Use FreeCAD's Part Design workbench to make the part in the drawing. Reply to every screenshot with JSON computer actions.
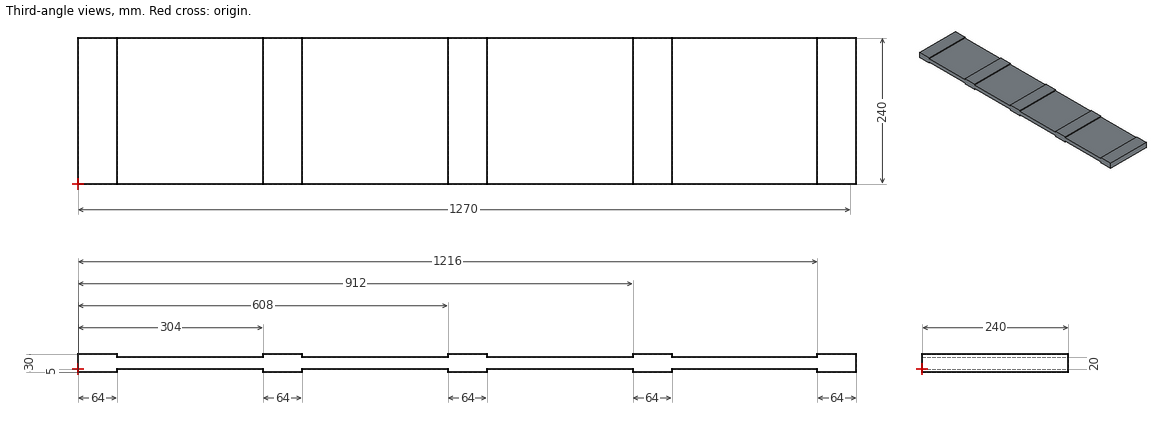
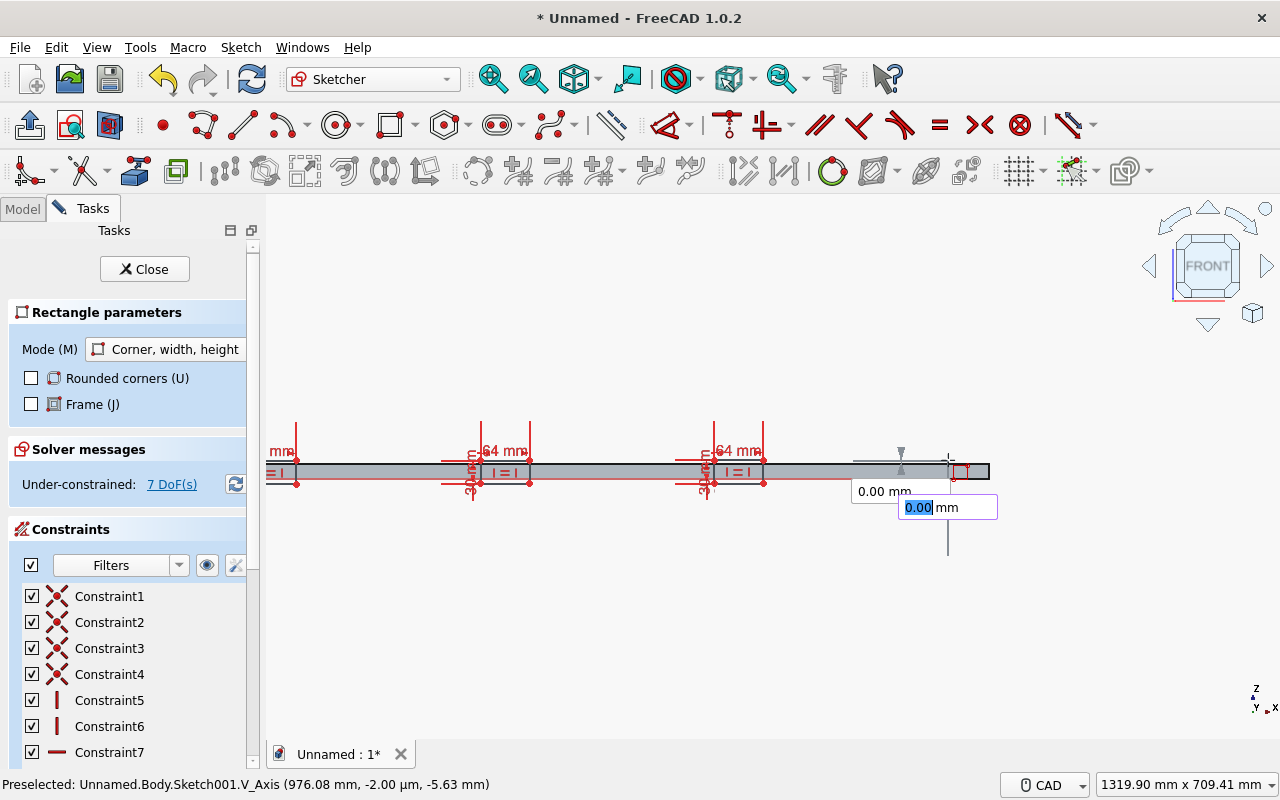
{"action": "scroll", "coordinate": [997, 483], "scroll_direction": "up", "scroll_amount": 8}
{"action": "mouse_move", "coordinate": [994, 481]}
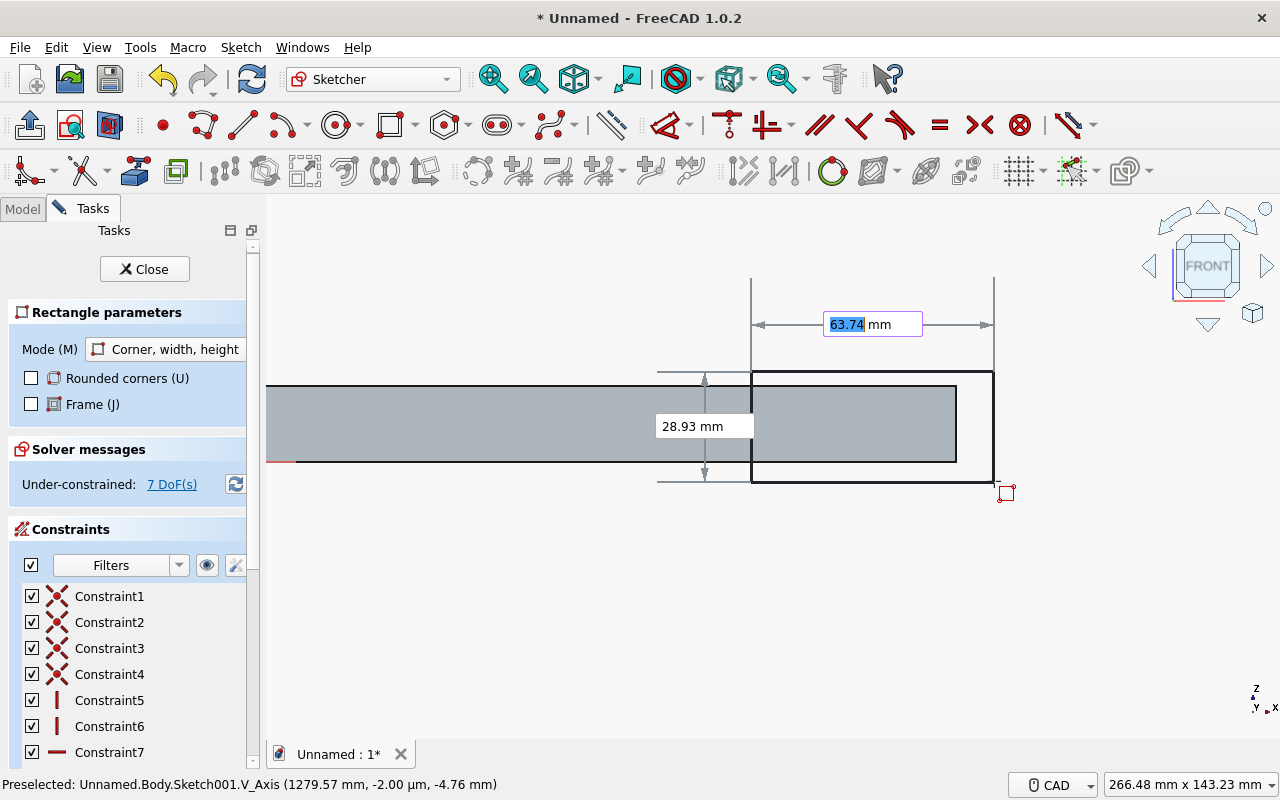
{"action": "type", "text": "64"}
{"action": "key", "text": "Tab"}
{"action": "type", "text": "30"}
{"action": "key", "text": "Return"}
{"action": "key", "text": "Escape"}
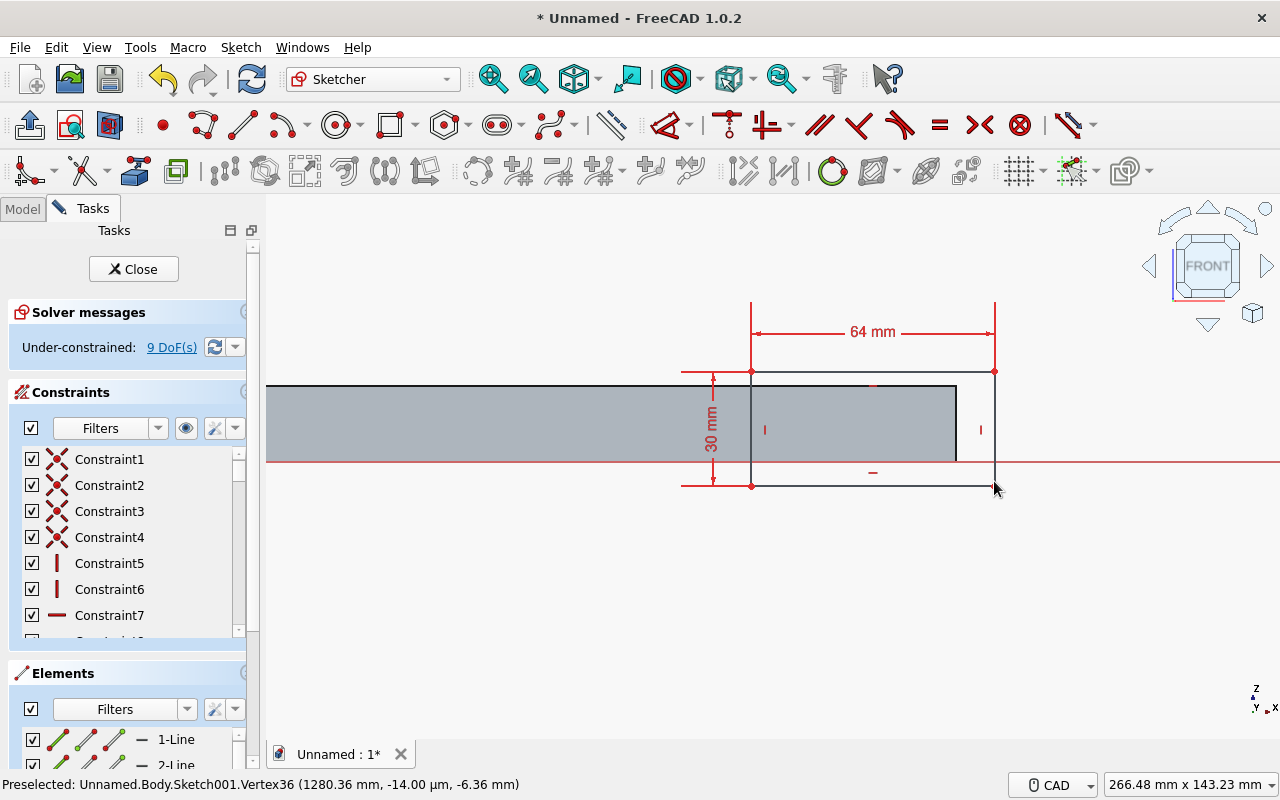
{"action": "key", "text": "d"}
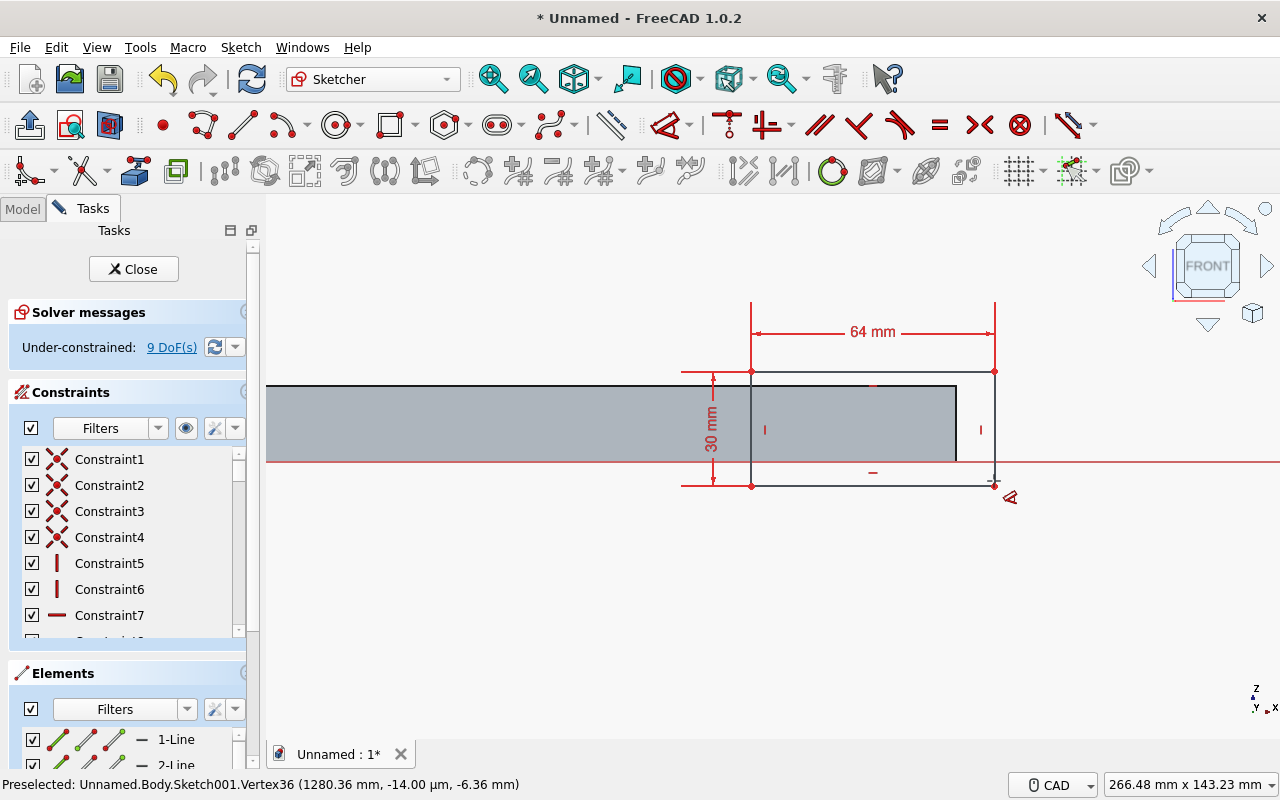
{"action": "scroll", "coordinate": [972, 472], "scroll_direction": "down", "scroll_amount": 11}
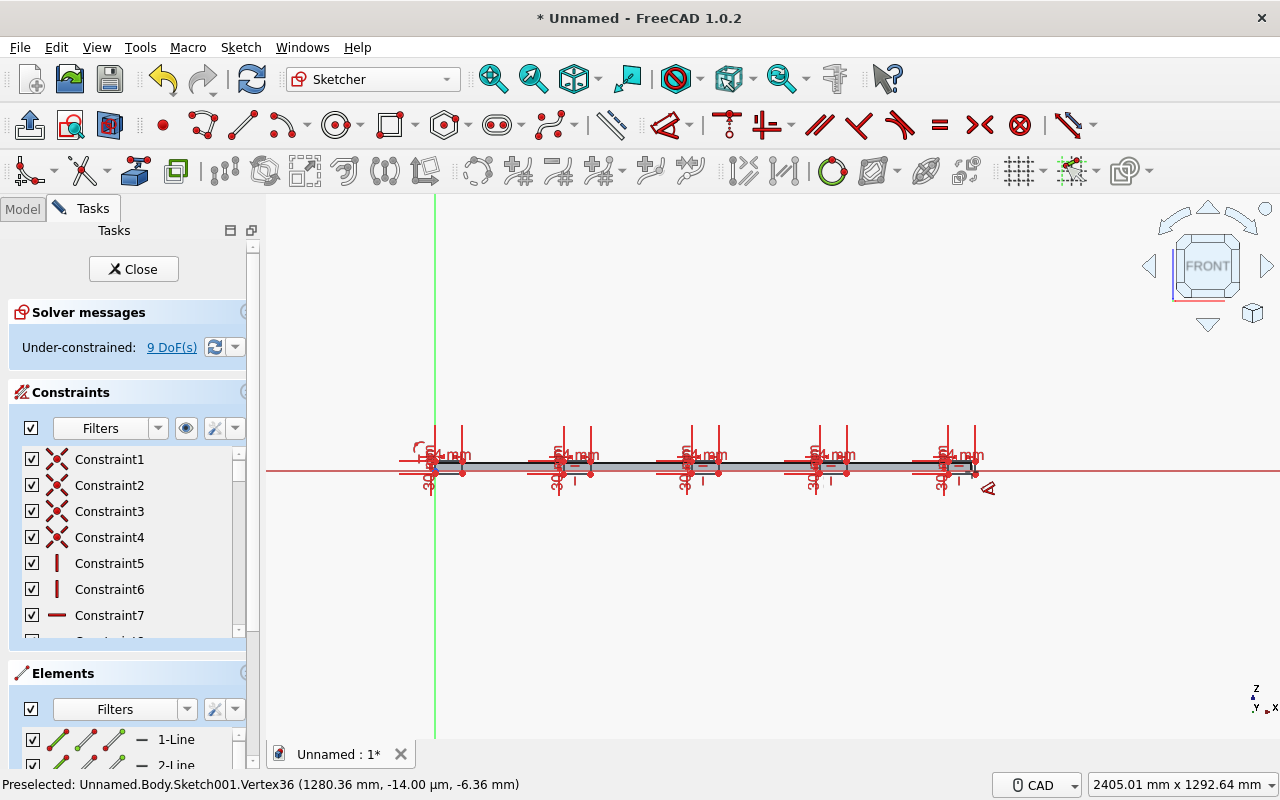
{"action": "scroll", "coordinate": [435, 474], "scroll_direction": "up", "scroll_amount": 15}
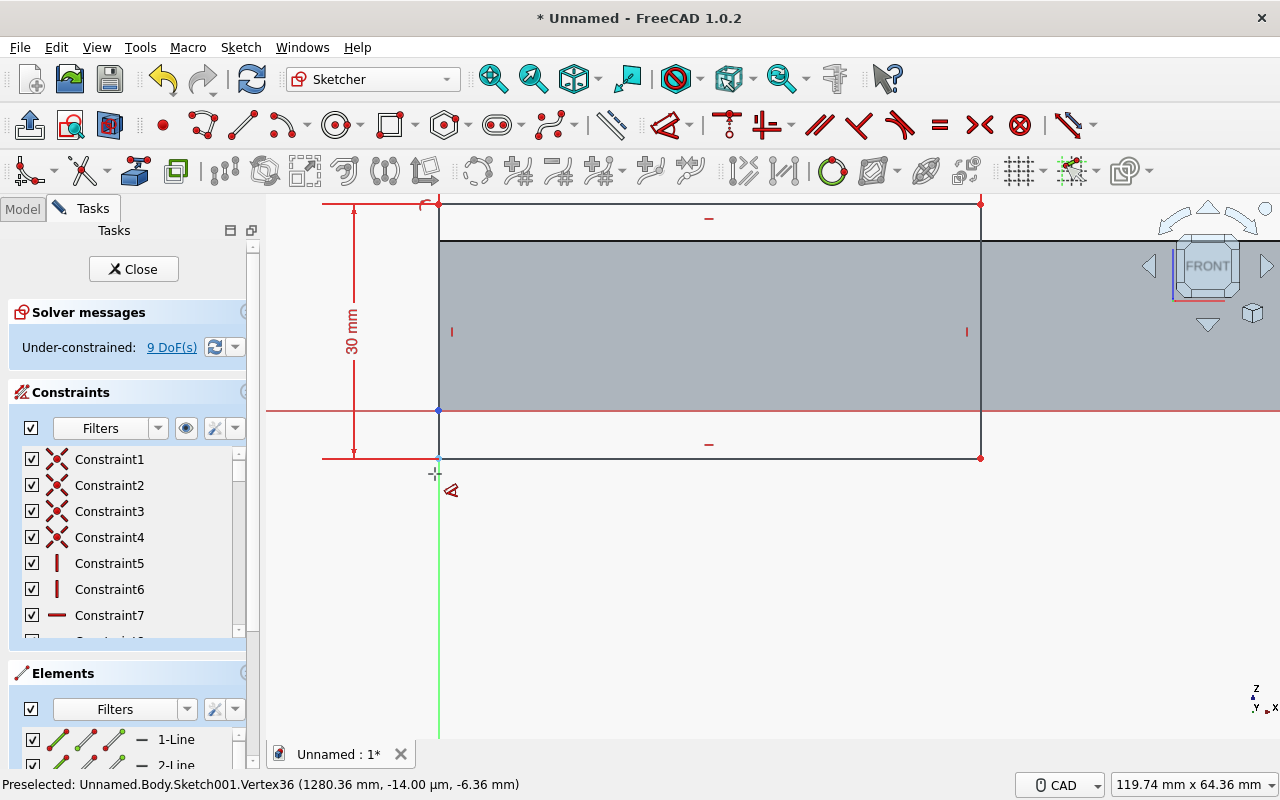
{"action": "left_click", "coordinate": [439, 459]}
{"action": "left_click", "coordinate": [405, 435]}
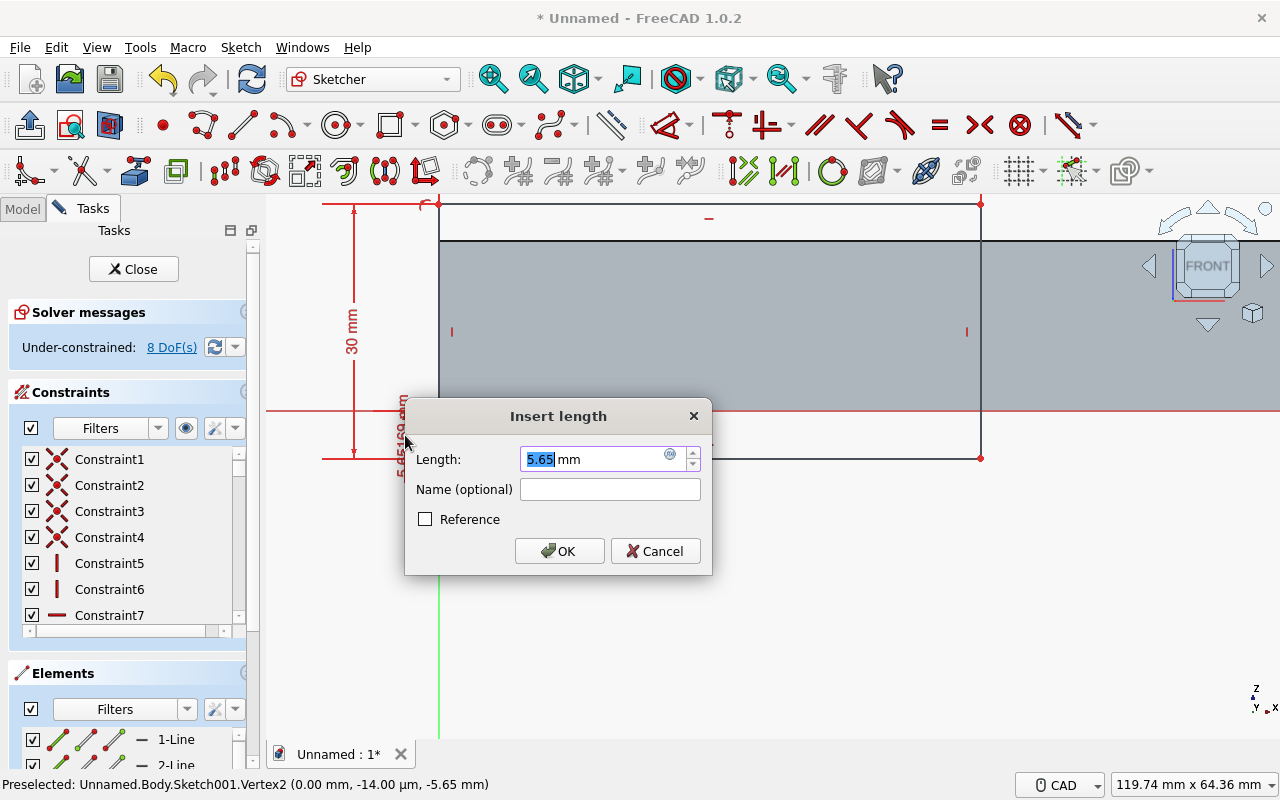
{"action": "type", "text": "5"}
{"action": "key", "text": "Return"}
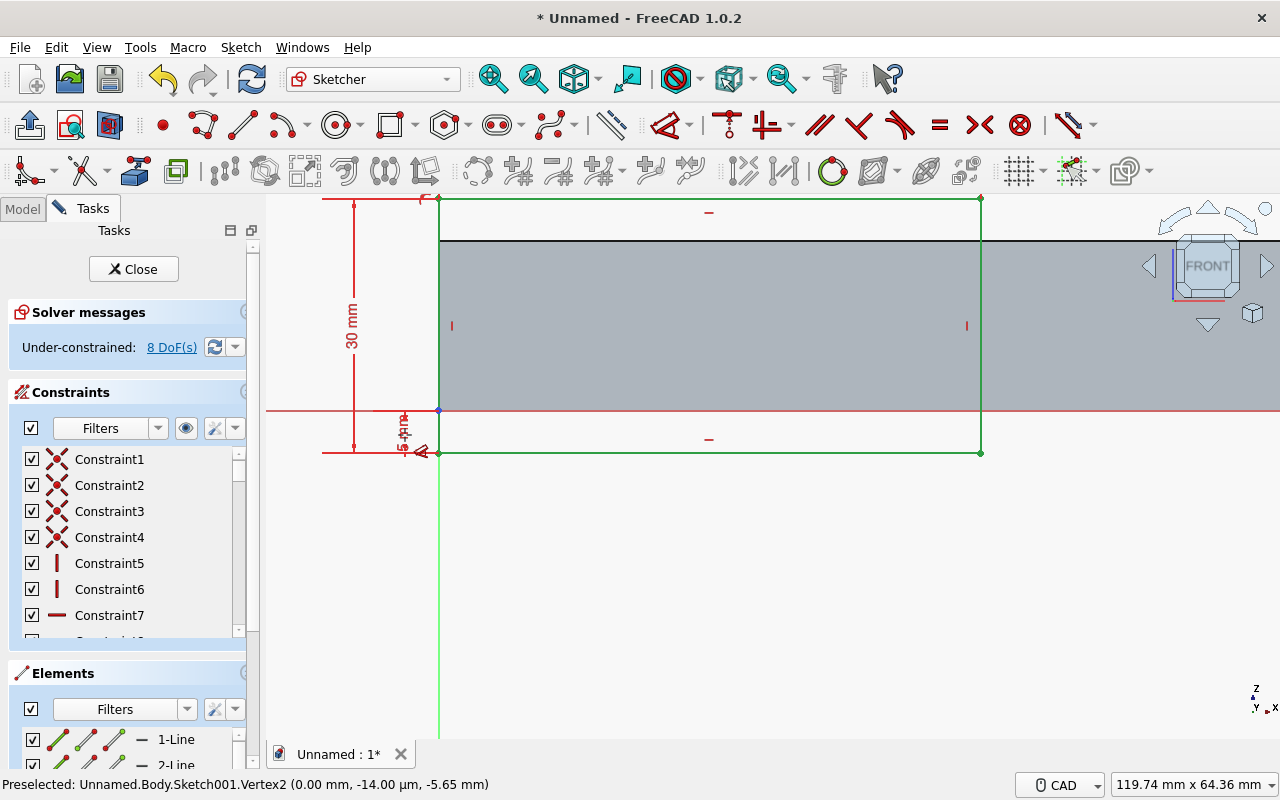
{"action": "scroll", "coordinate": [434, 474], "scroll_direction": "down", "scroll_amount": 15}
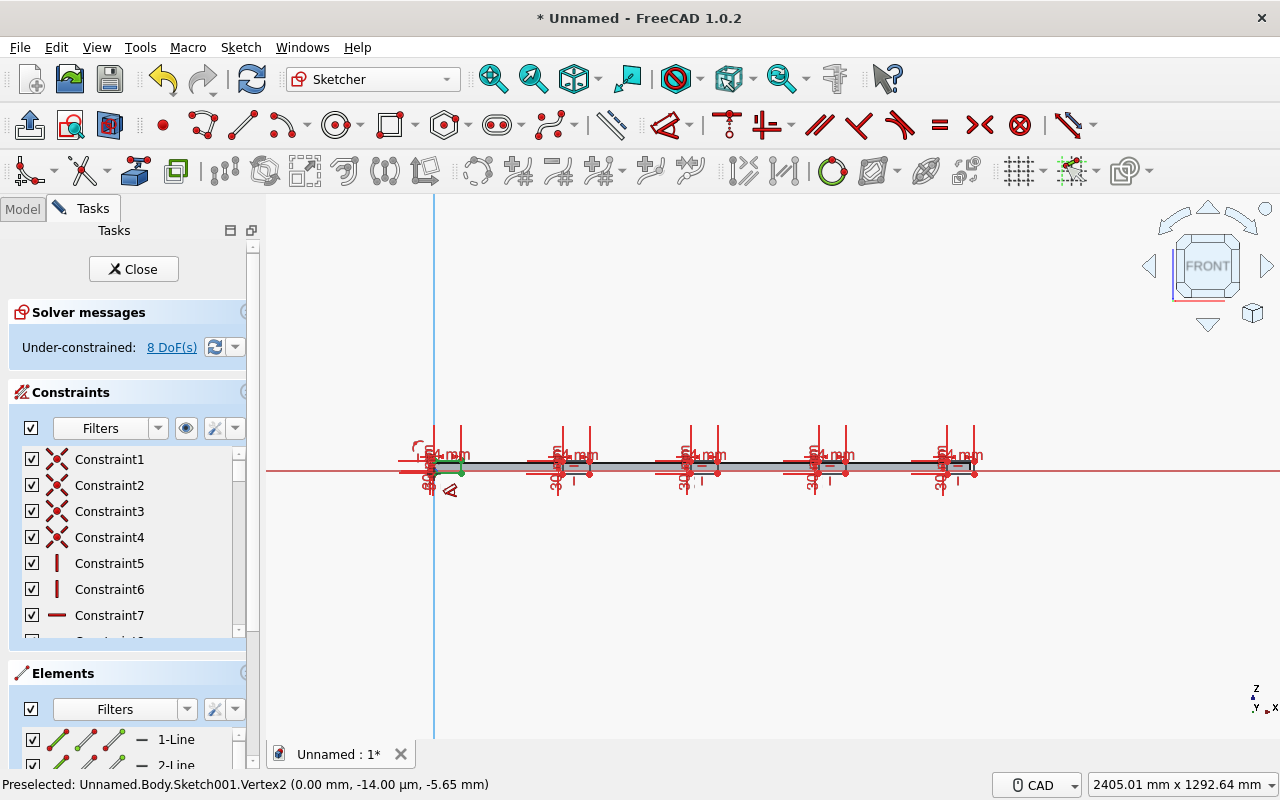
{"action": "scroll", "coordinate": [563, 474], "scroll_direction": "up", "scroll_amount": 15}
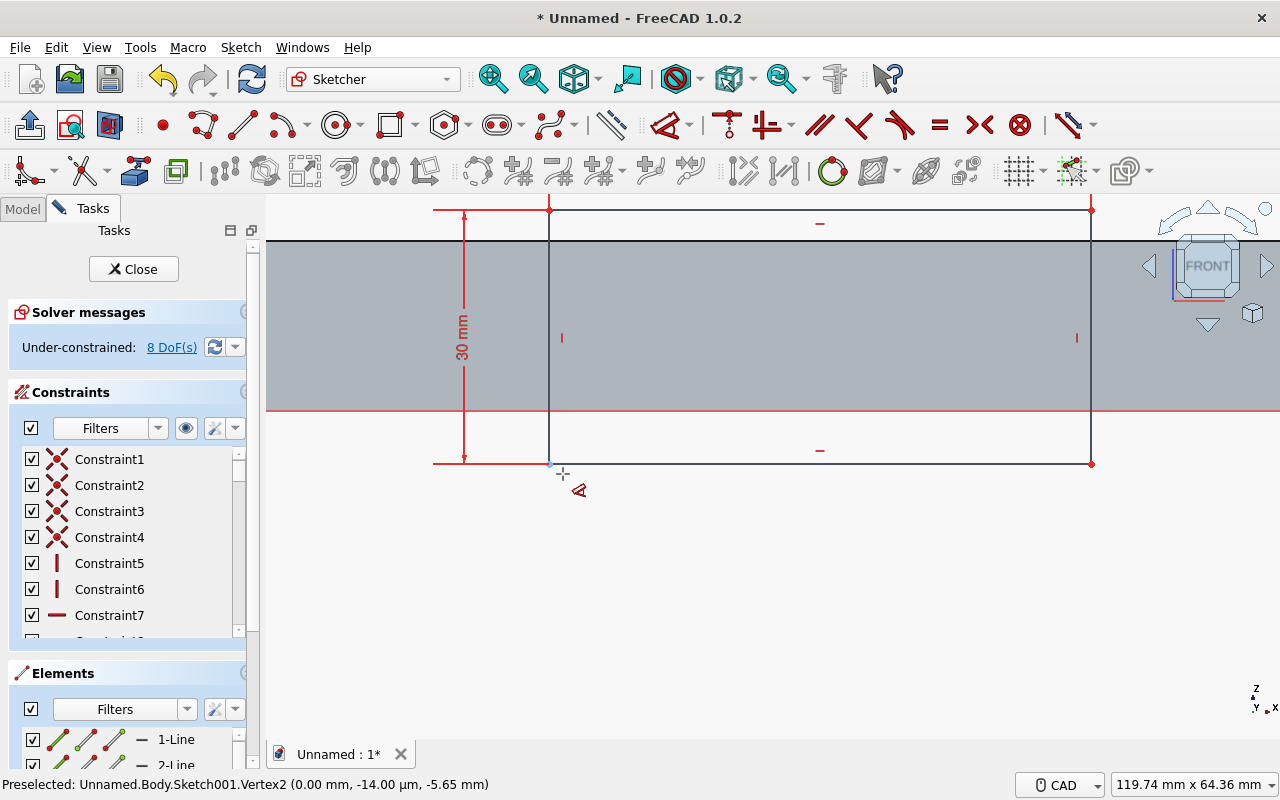
{"action": "left_click", "coordinate": [549, 464]}
{"action": "left_click", "coordinate": [583, 438]}